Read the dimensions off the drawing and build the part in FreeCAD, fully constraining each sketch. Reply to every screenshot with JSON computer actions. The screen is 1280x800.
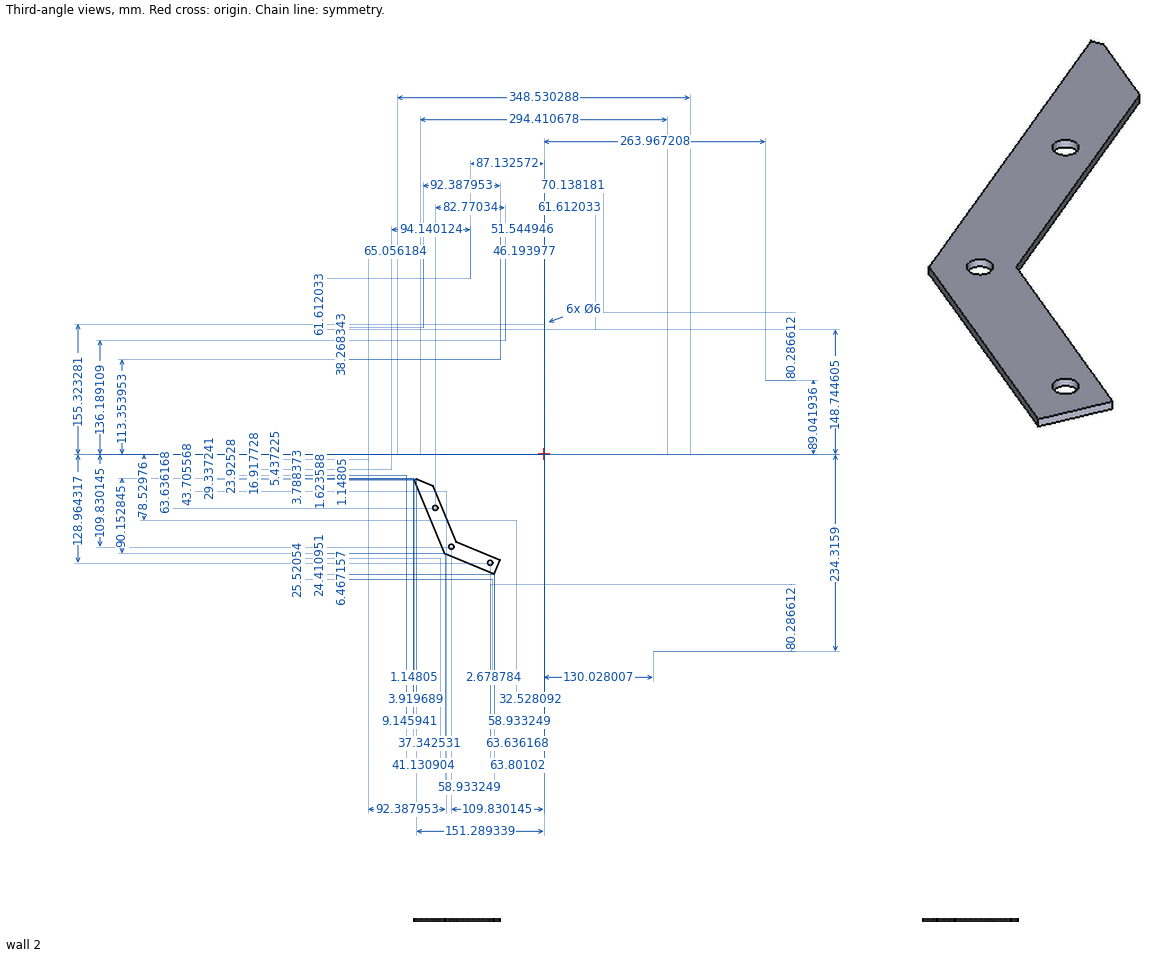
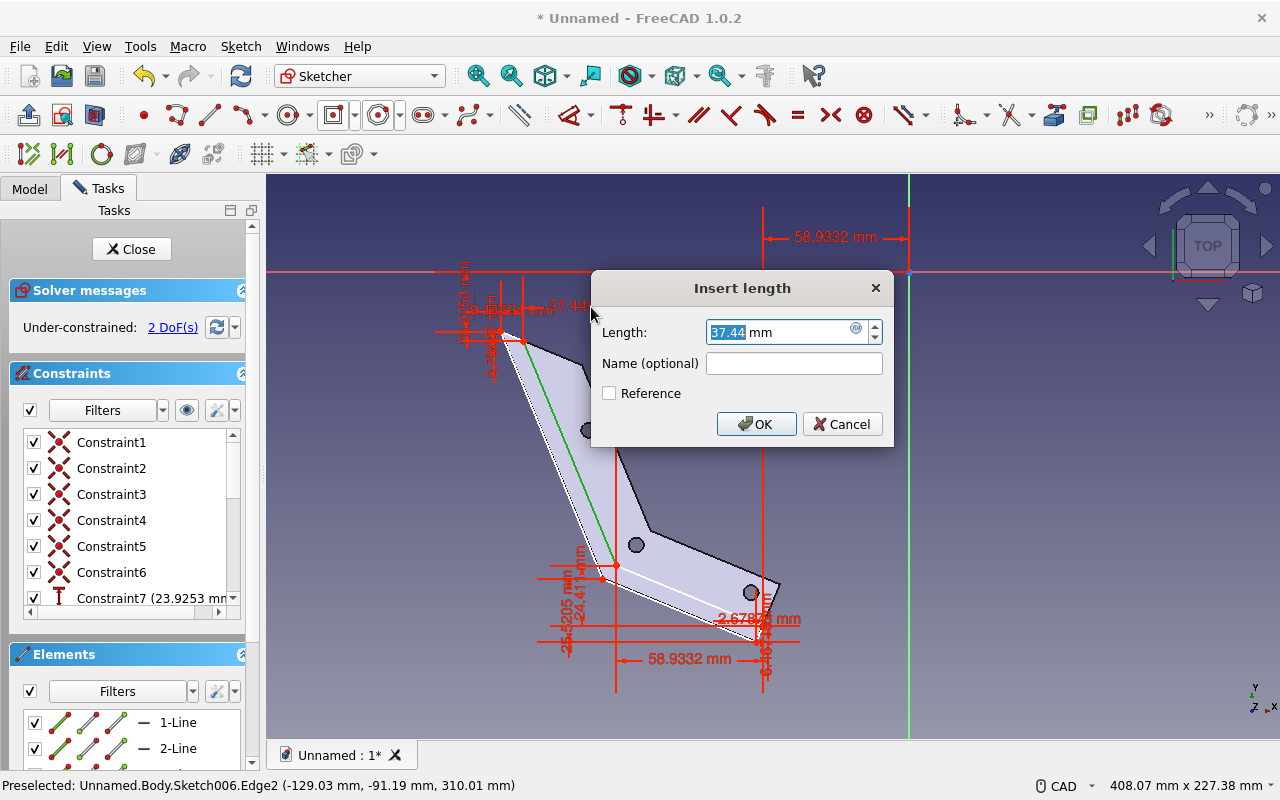
{"action": "type", "text": "37.342531"}
{"action": "key", "text": "Return"}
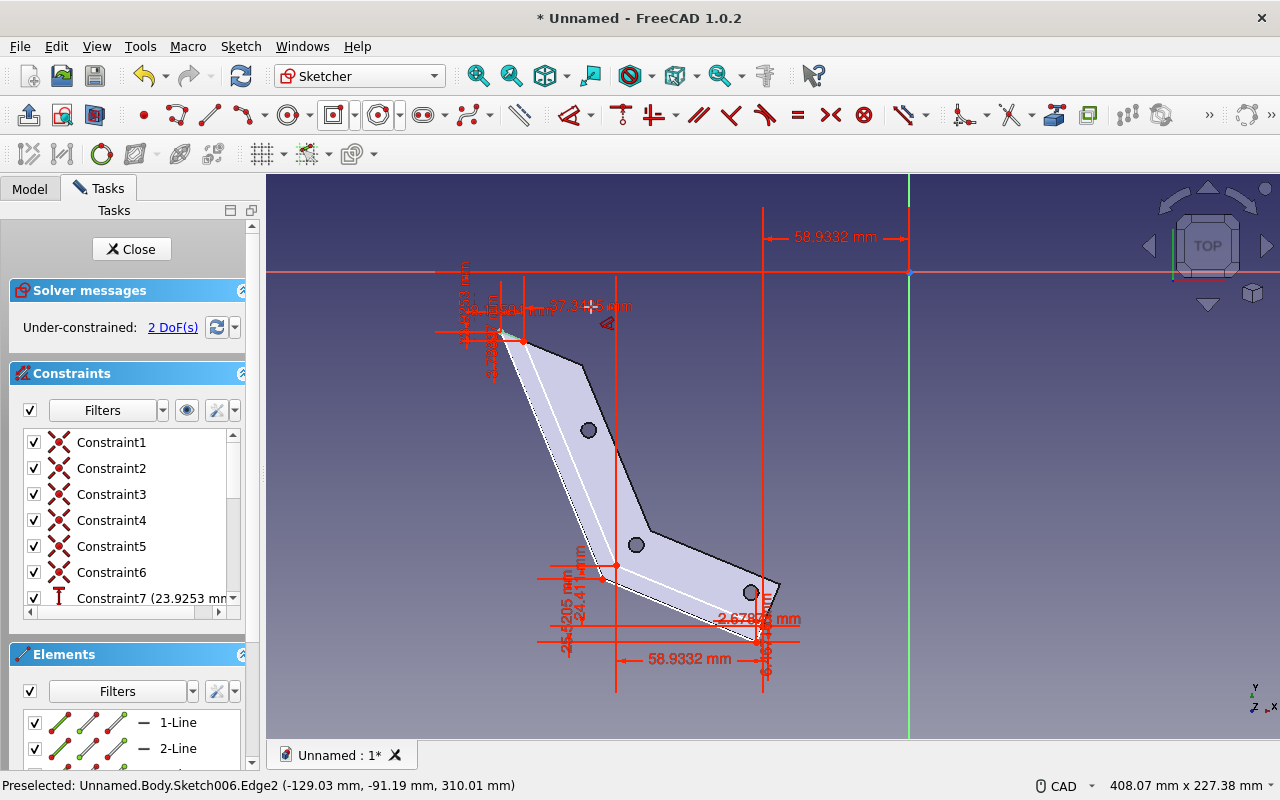
{"action": "left_click", "coordinate": [589, 498]}
{"action": "left_click", "coordinate": [490, 453]}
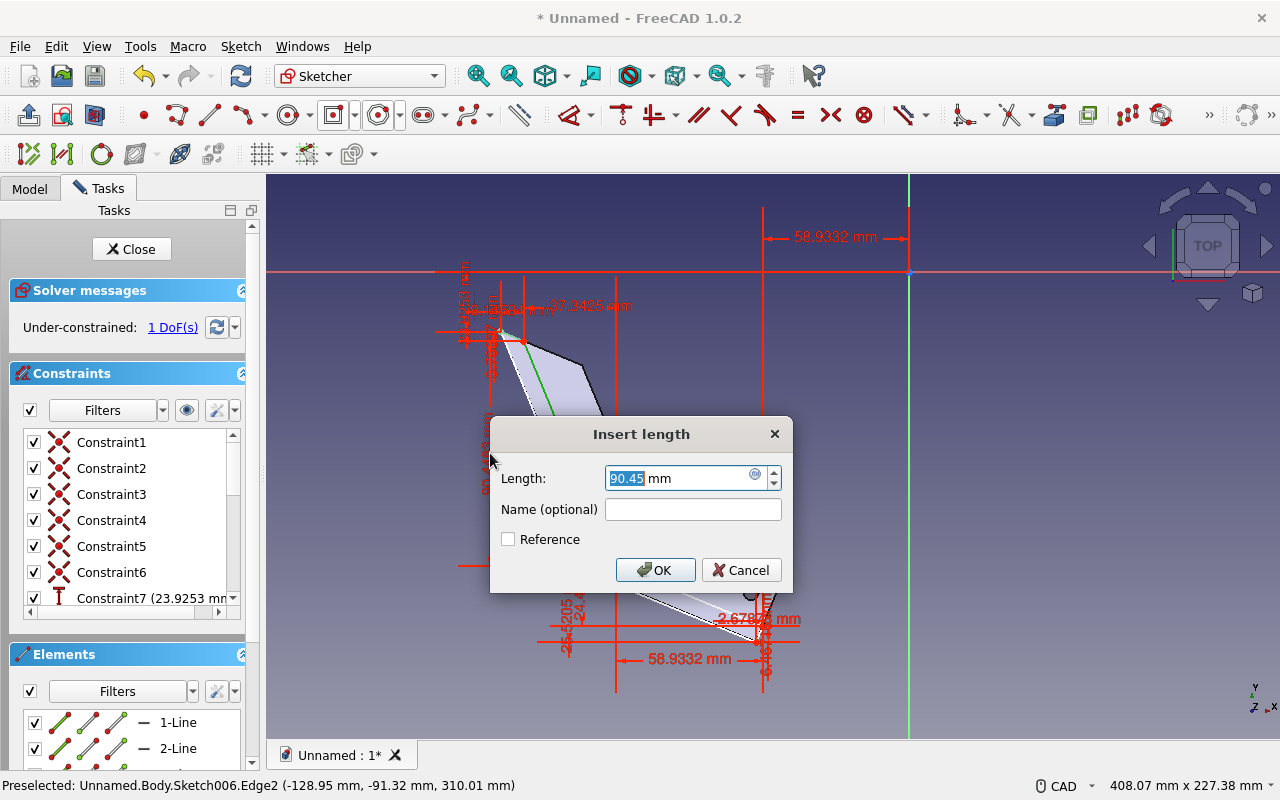
{"action": "type", "text": "90.152845"}
{"action": "key", "text": "Return"}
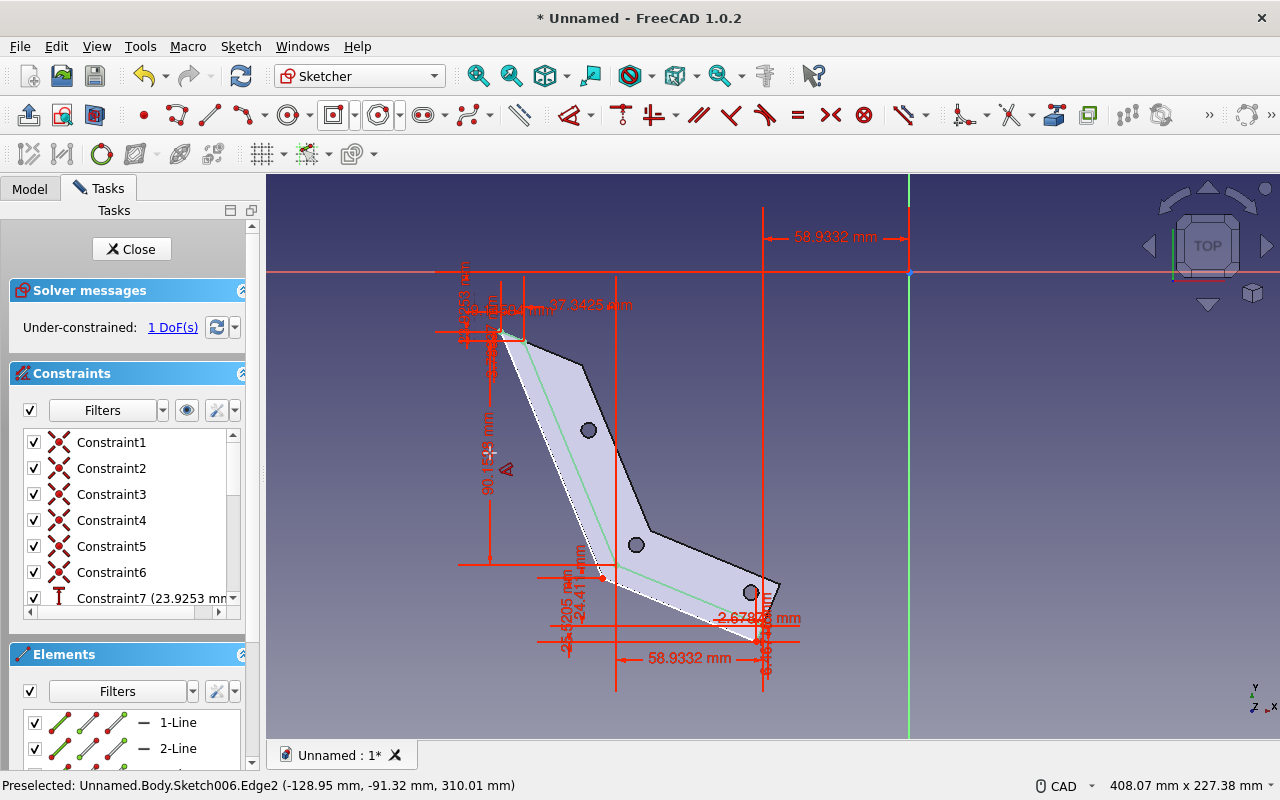
{"action": "left_click", "coordinate": [531, 406]}
{"action": "left_click", "coordinate": [552, 636]}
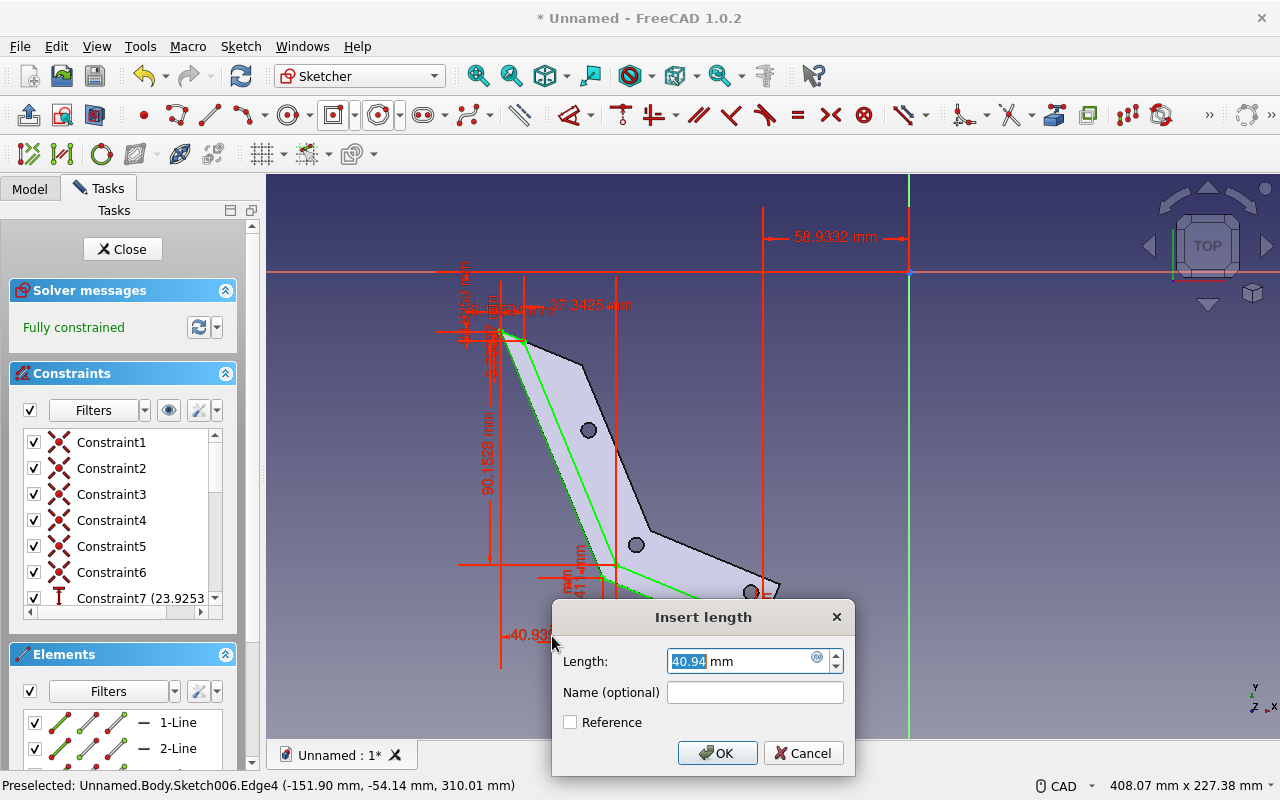
{"action": "type", "text": "41.130904"}
{"action": "key", "text": "Return"}
{"action": "key", "text": "Escape"}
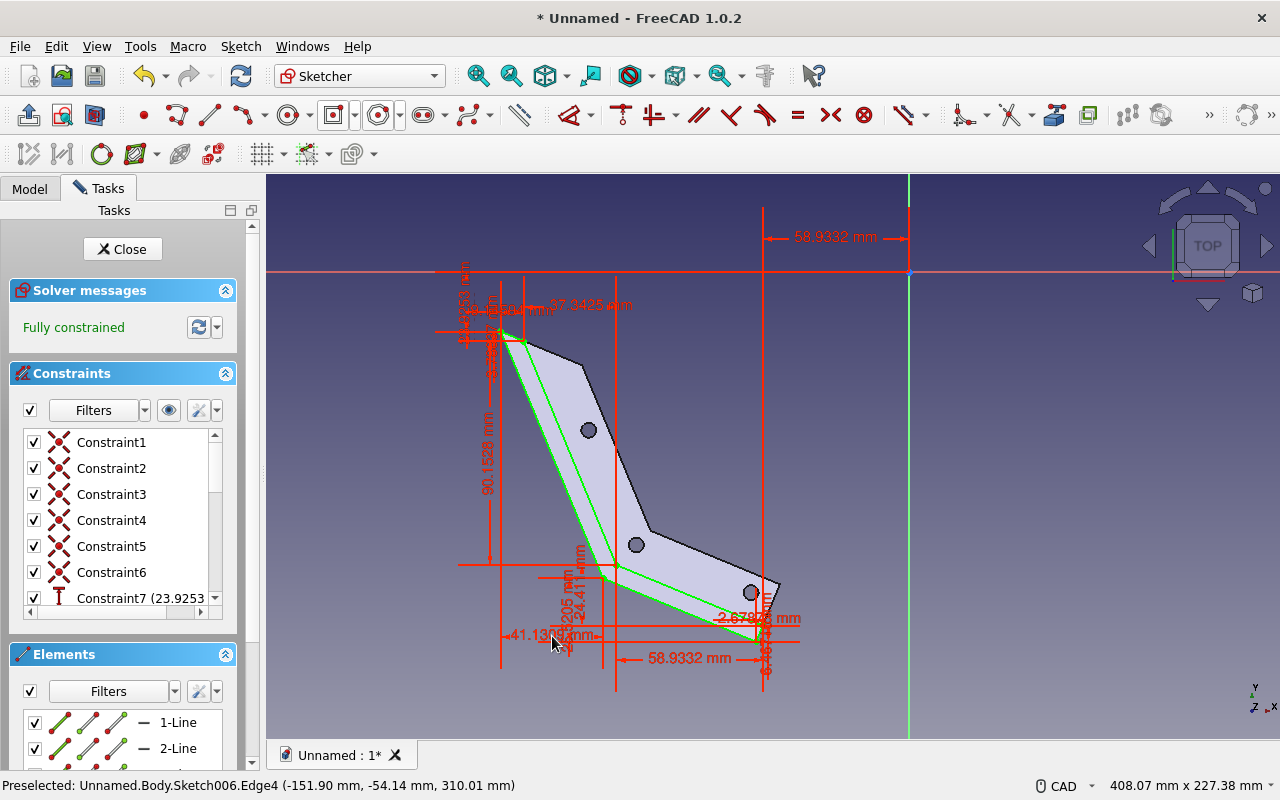
{"action": "left_click", "coordinate": [123, 249]}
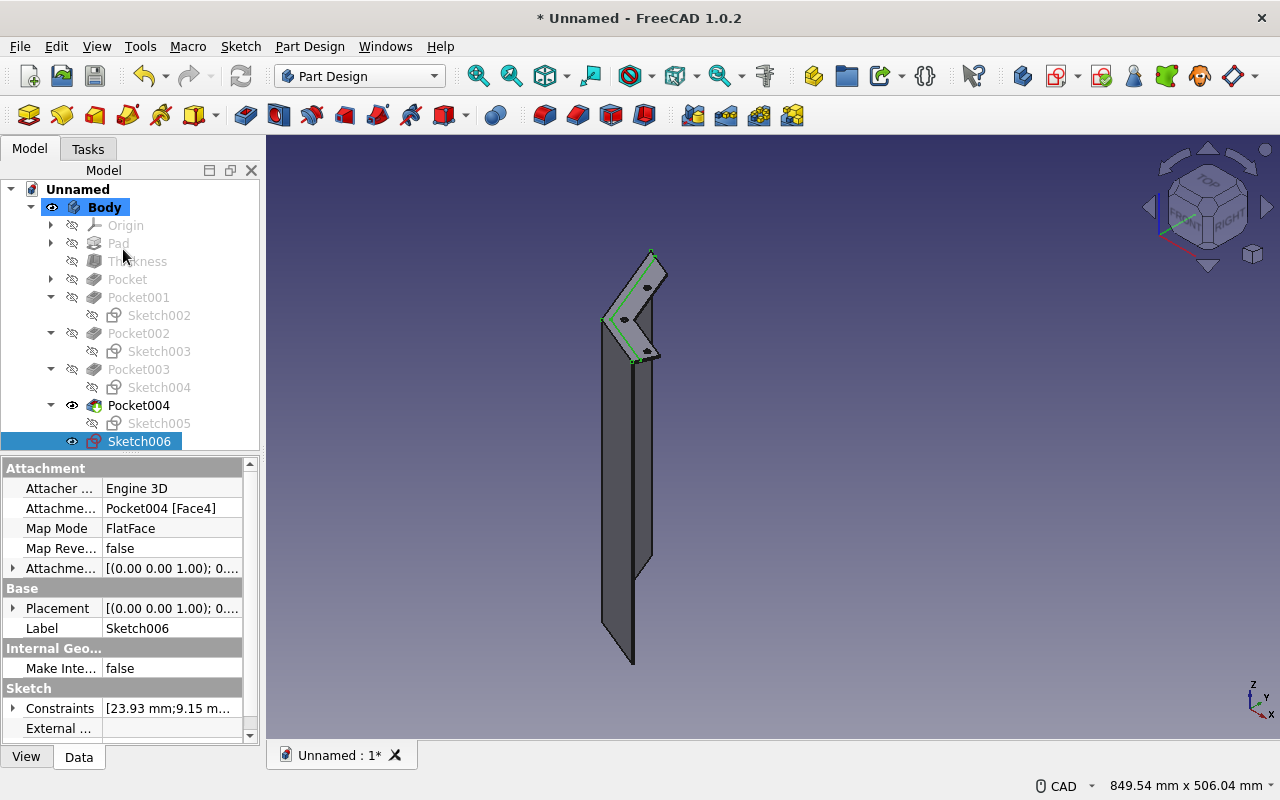
{"action": "left_click", "coordinate": [246, 116]}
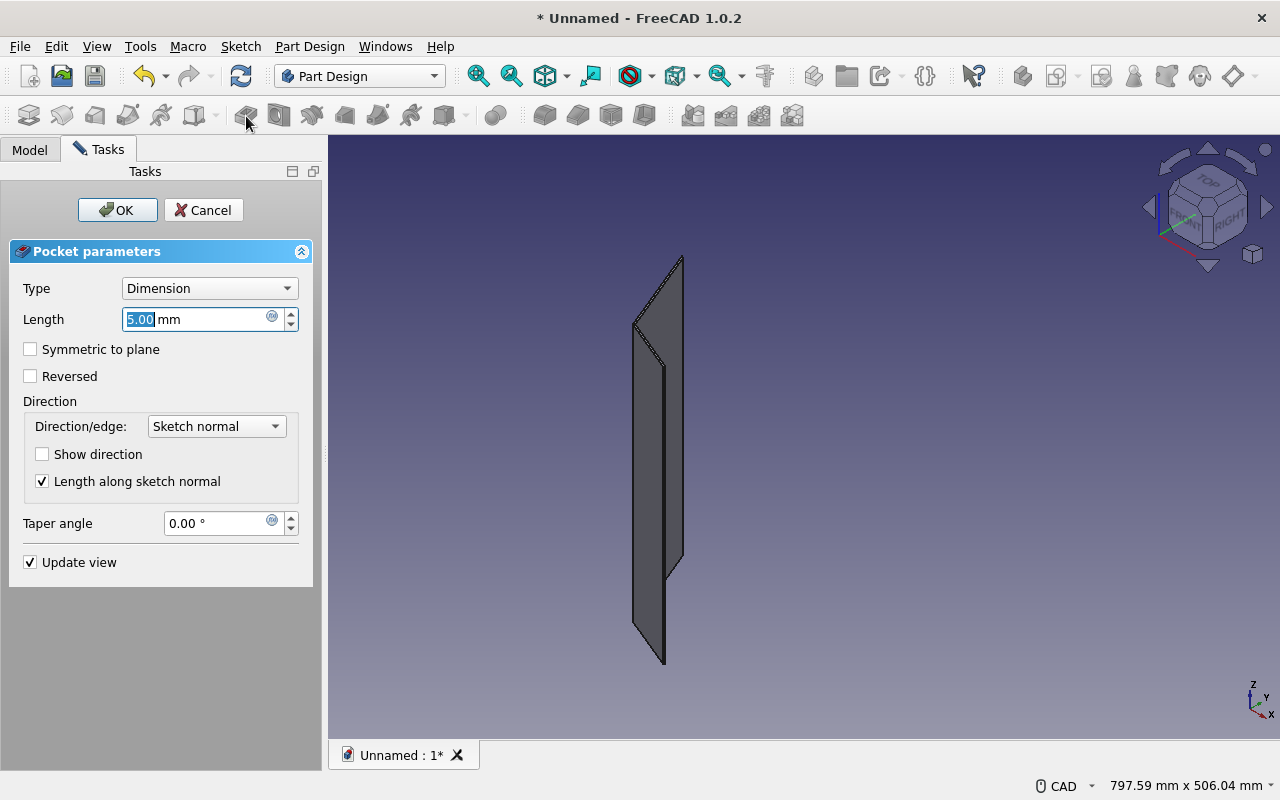
{"action": "left_click", "coordinate": [210, 288]}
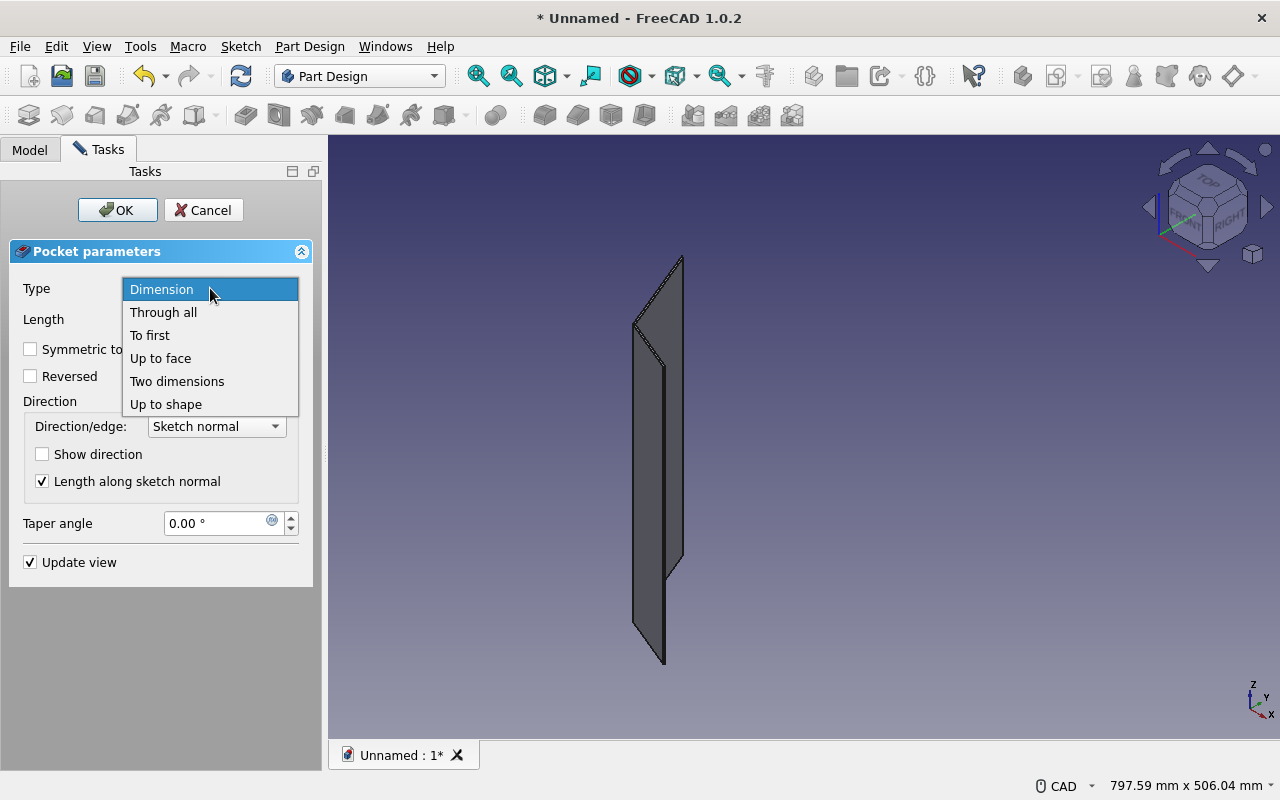
{"action": "left_click", "coordinate": [208, 312]}